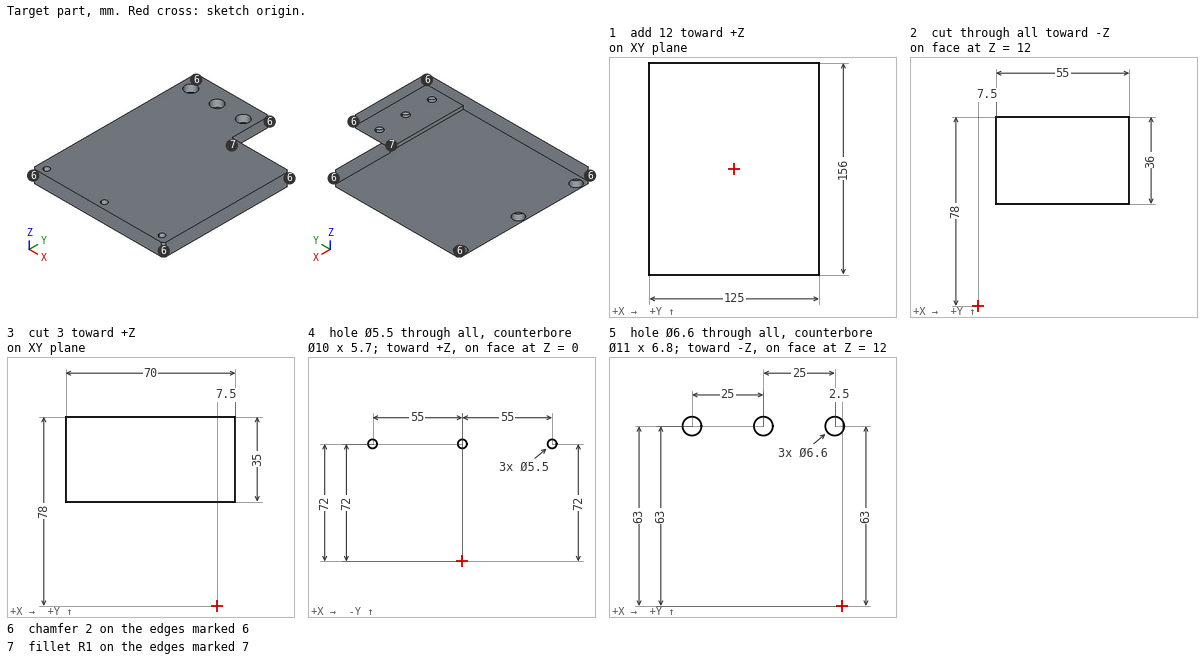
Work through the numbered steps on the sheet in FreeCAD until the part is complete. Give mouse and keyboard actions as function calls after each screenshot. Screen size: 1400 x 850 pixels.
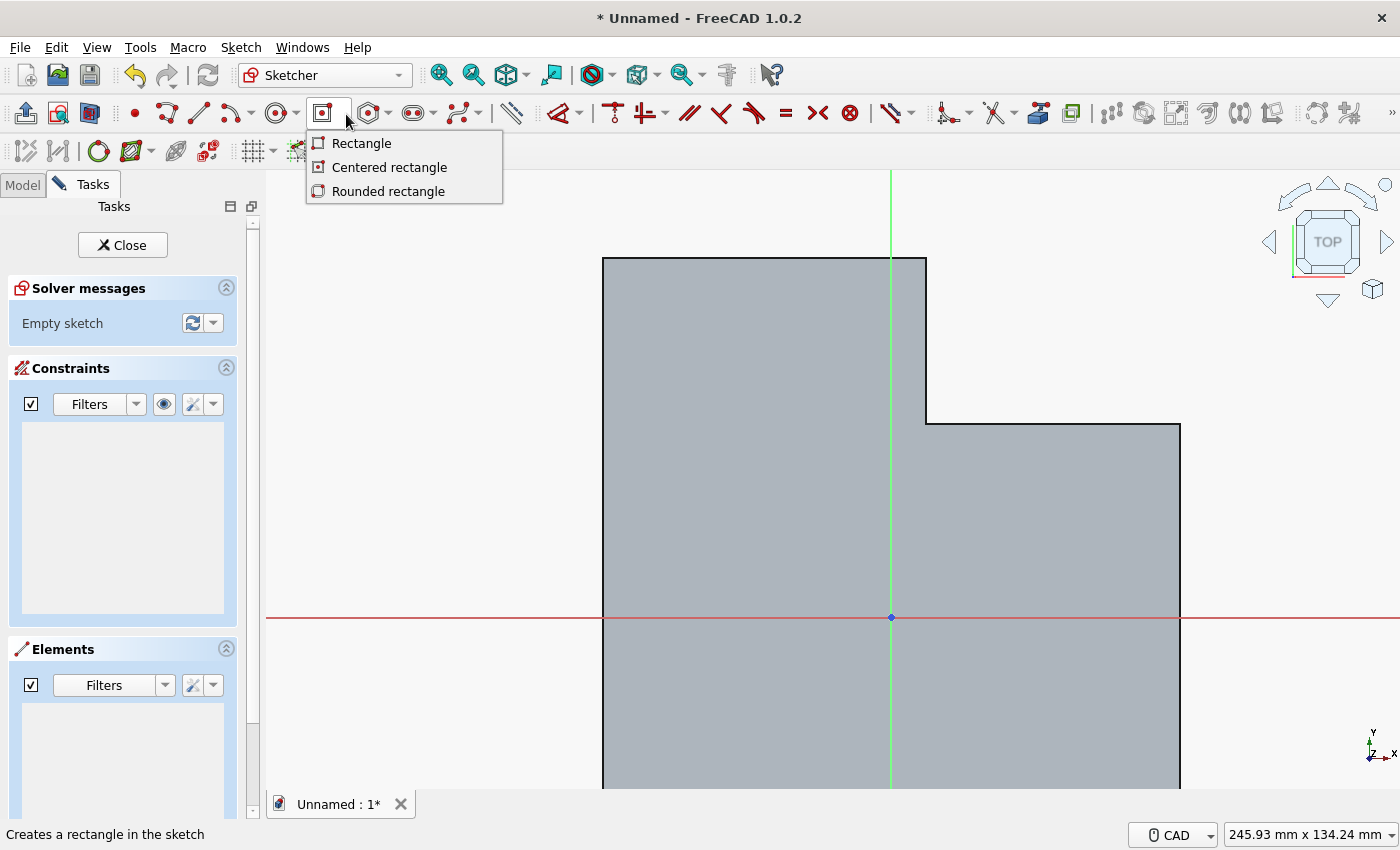
click(404, 143)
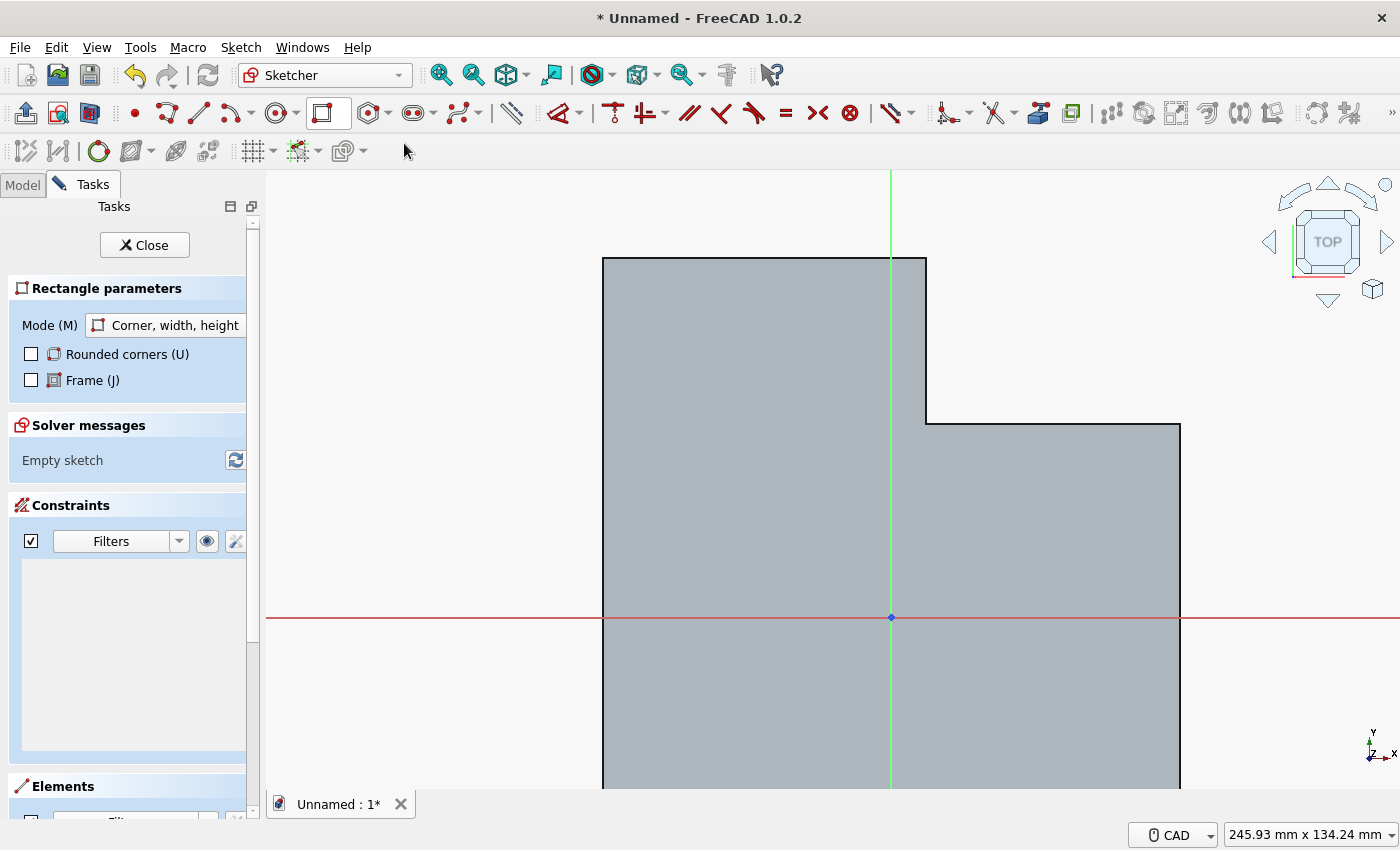
click(603, 258)
move(926, 420)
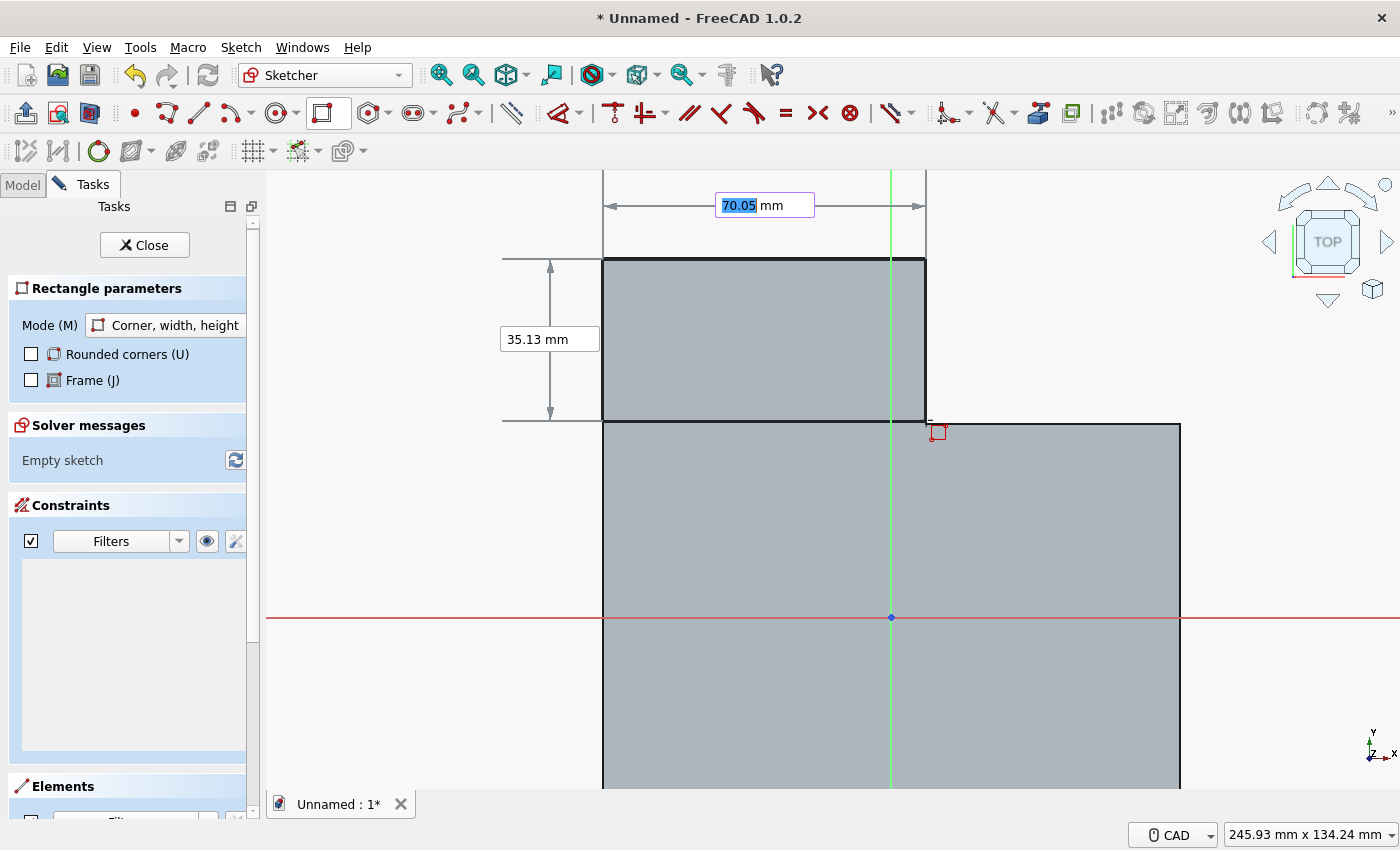
text(70)
key(Tab)
text(35)
key(Return)
key(Escape)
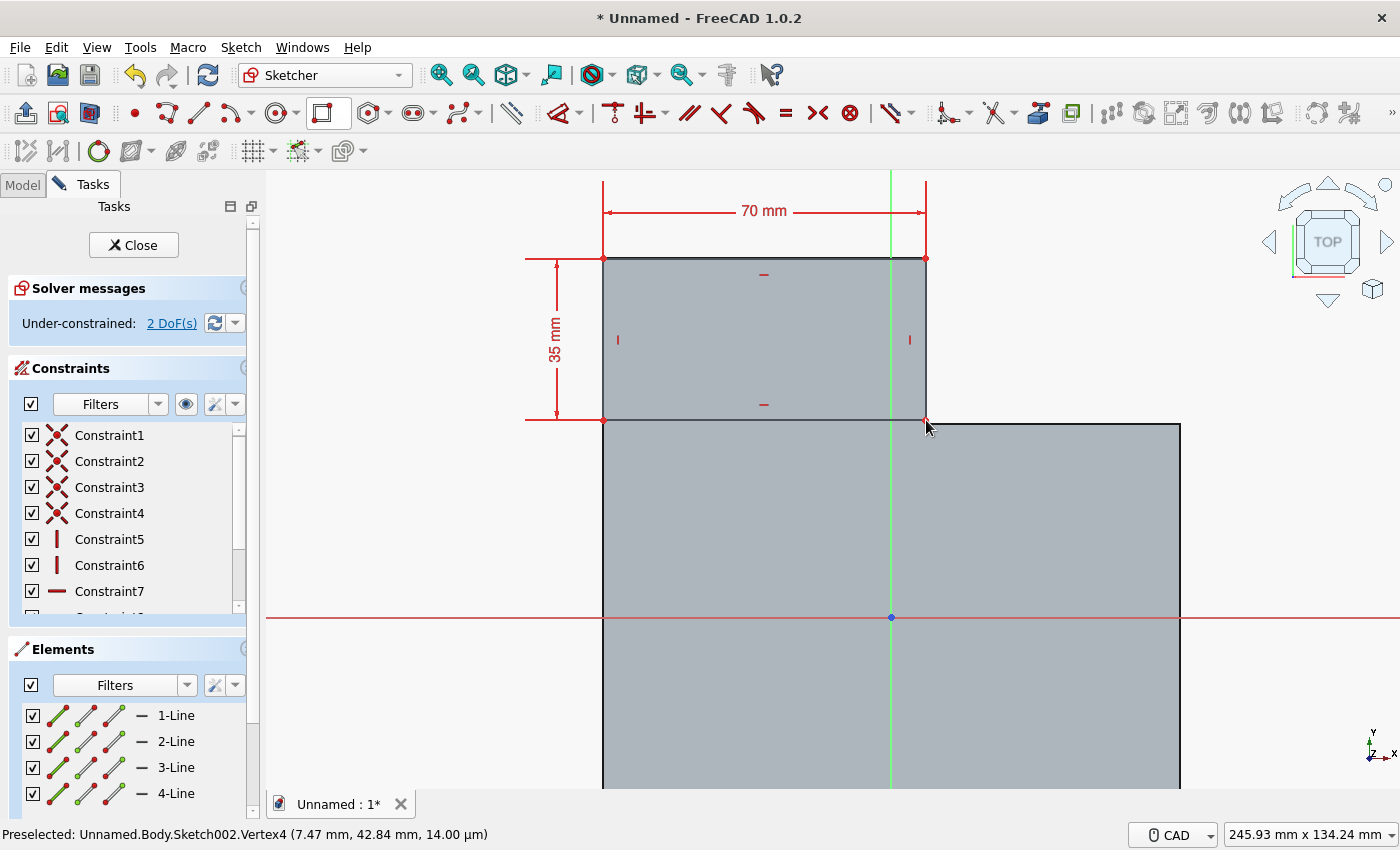
click(558, 114)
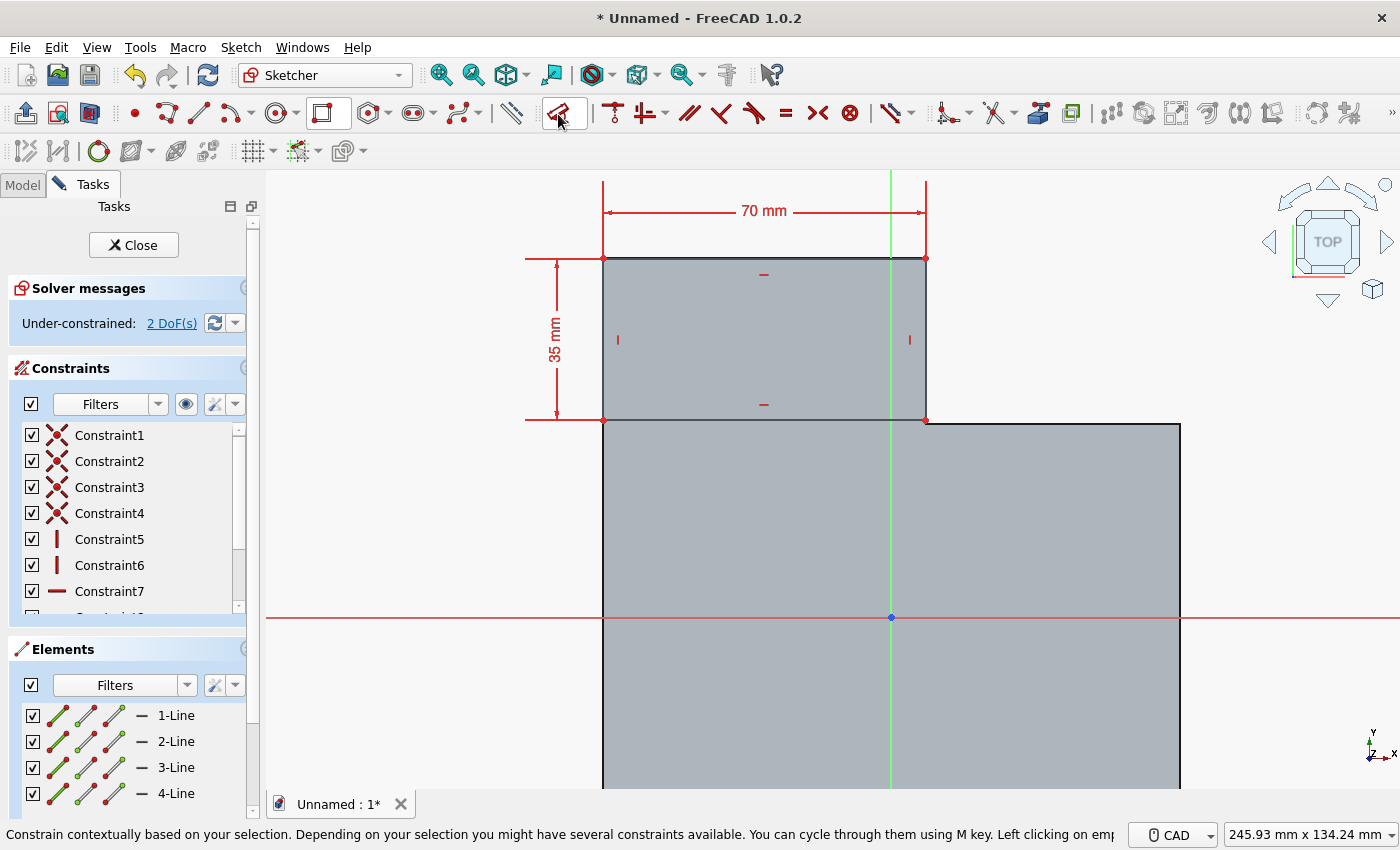
click(603, 259)
click(569, 438)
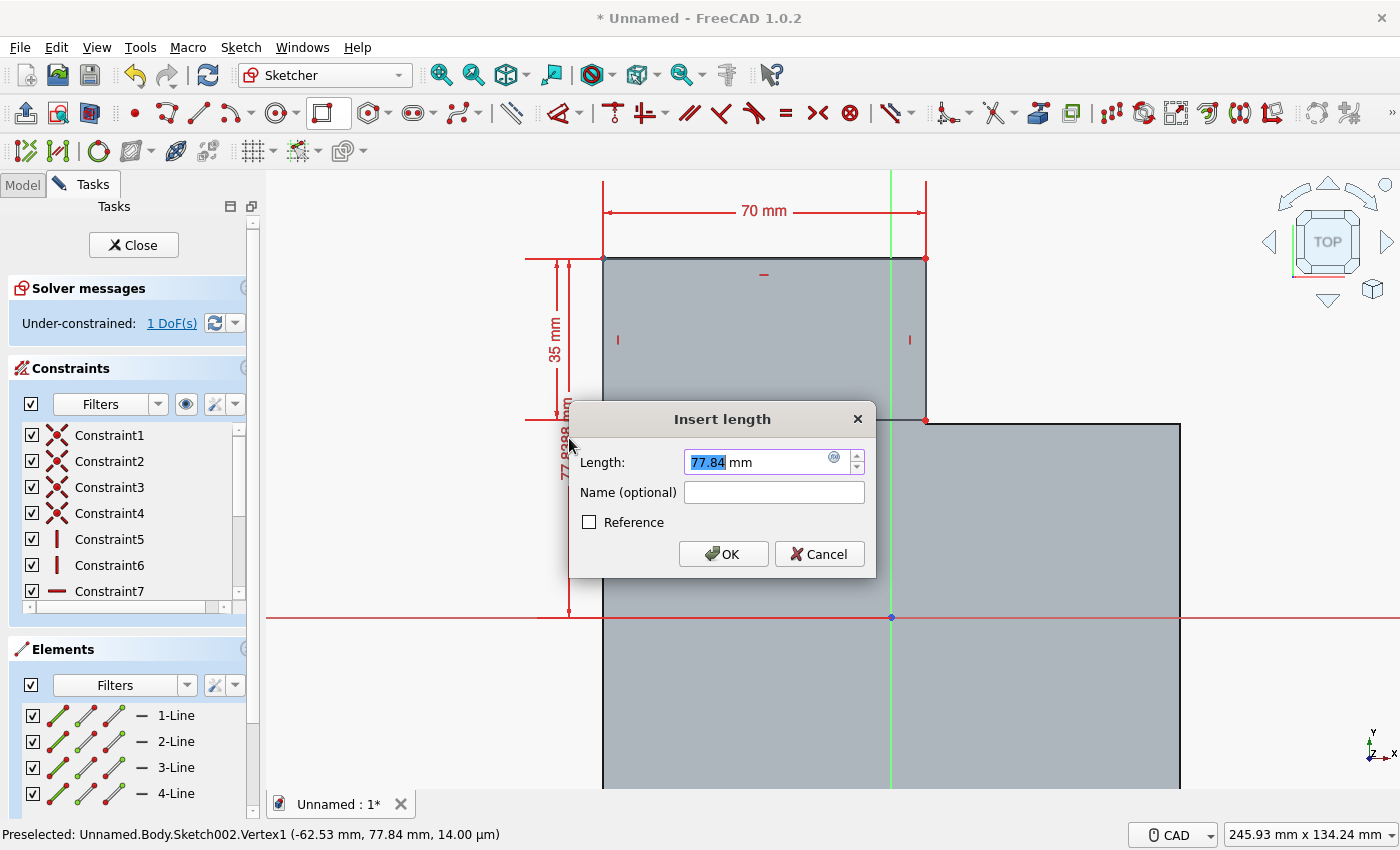
text(78)
key(Return)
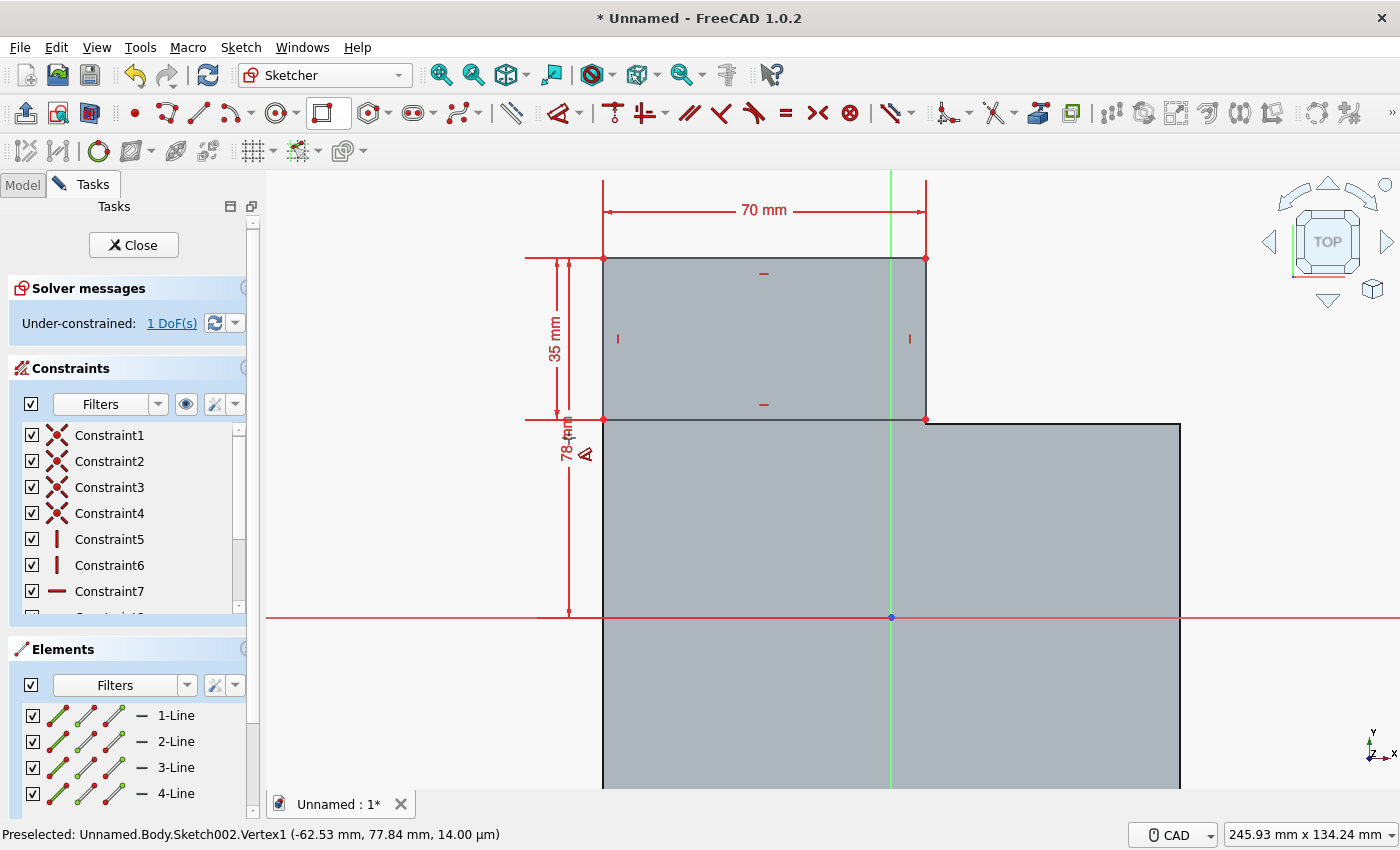
click(926, 420)
click(909, 652)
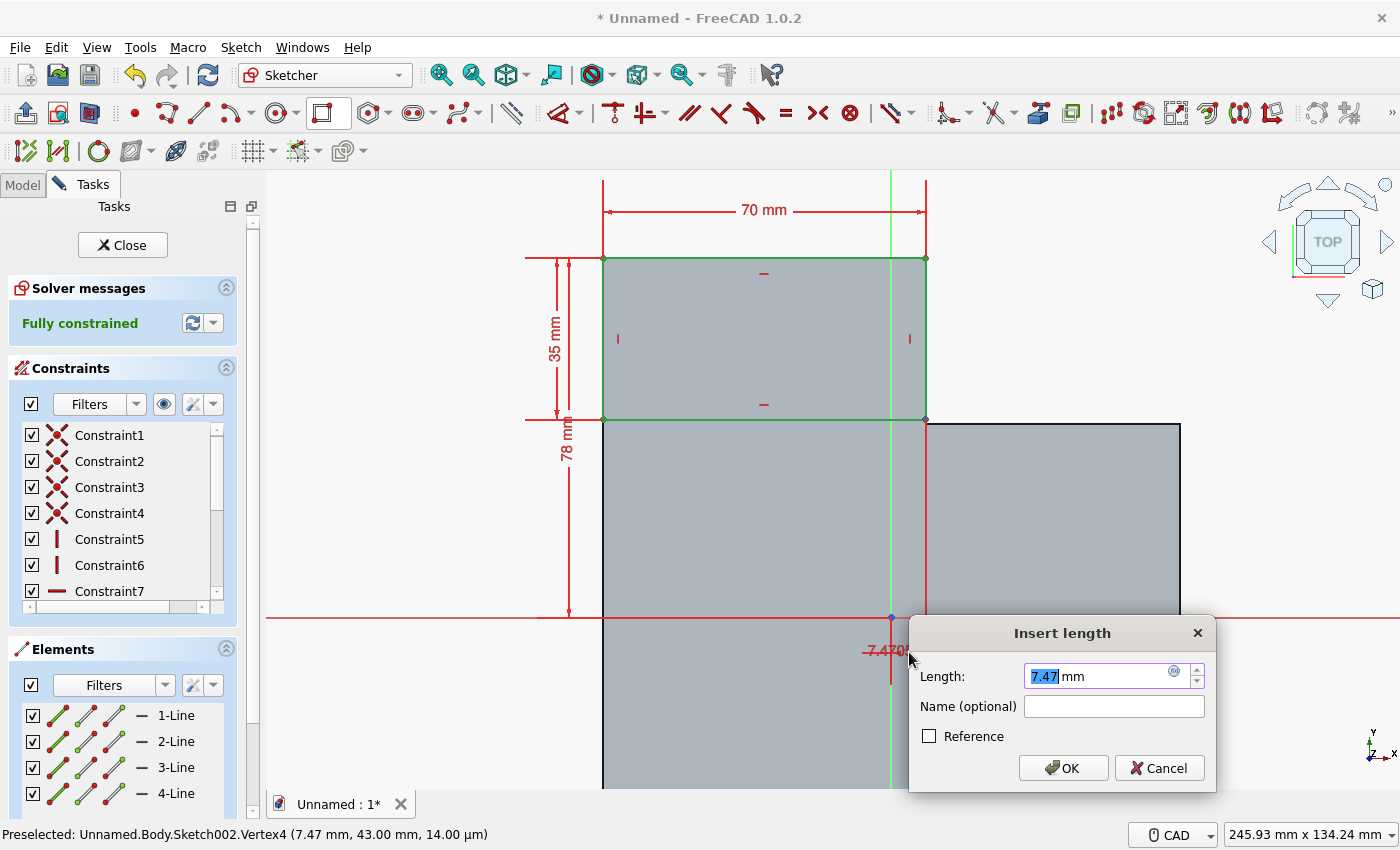
text(7.5)
key(Return)
key(Escape)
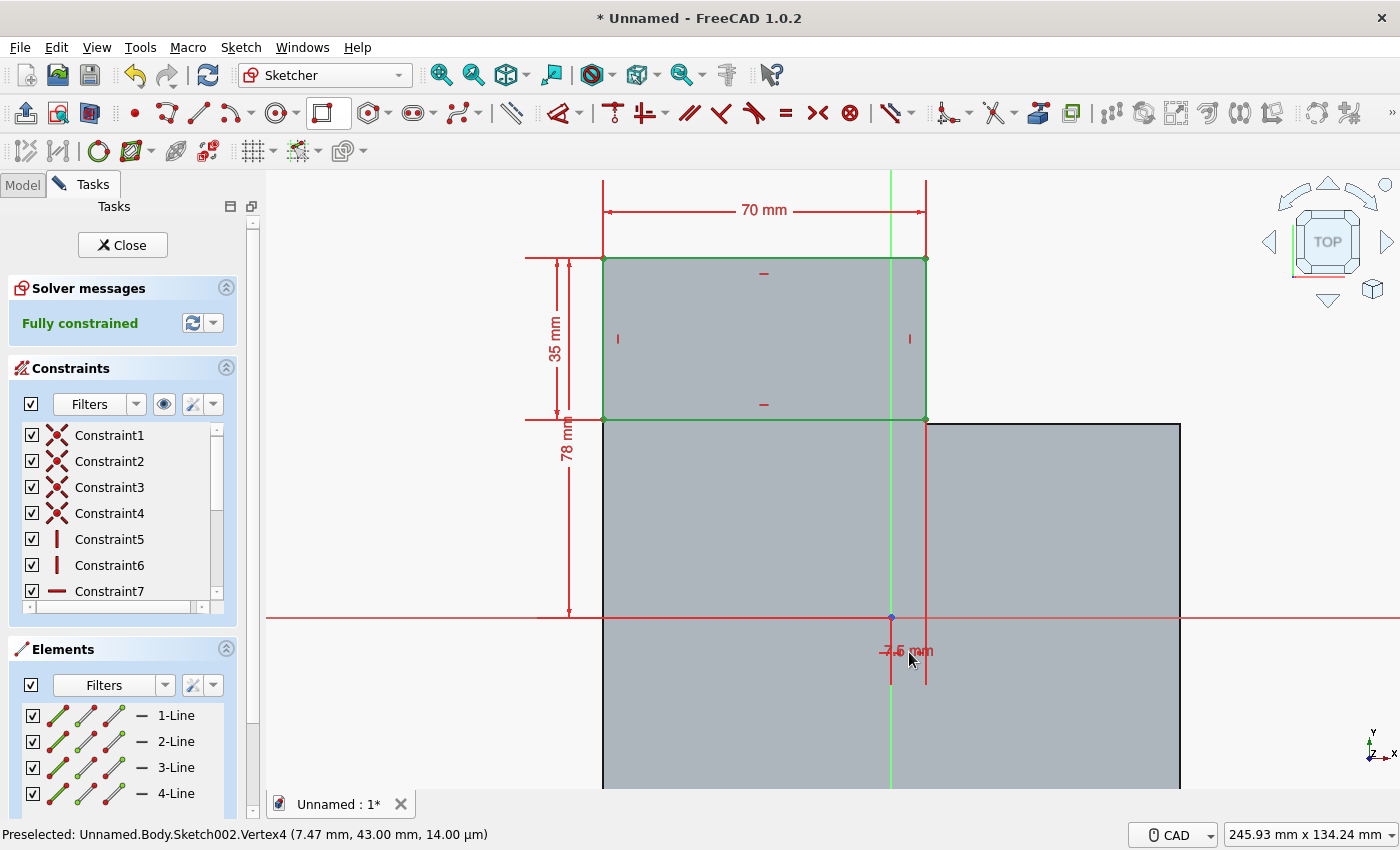
click(123, 245)